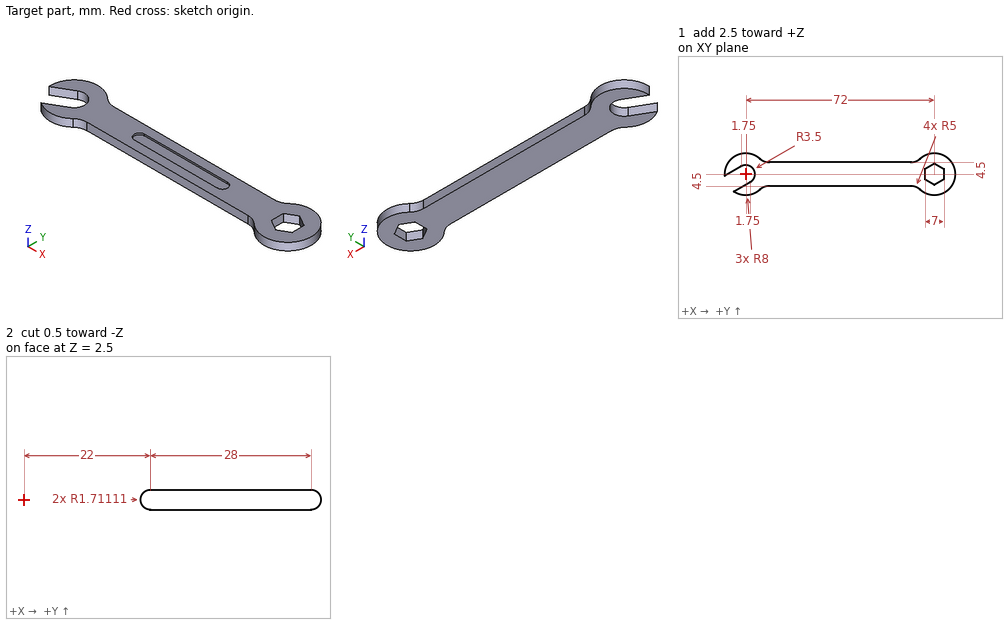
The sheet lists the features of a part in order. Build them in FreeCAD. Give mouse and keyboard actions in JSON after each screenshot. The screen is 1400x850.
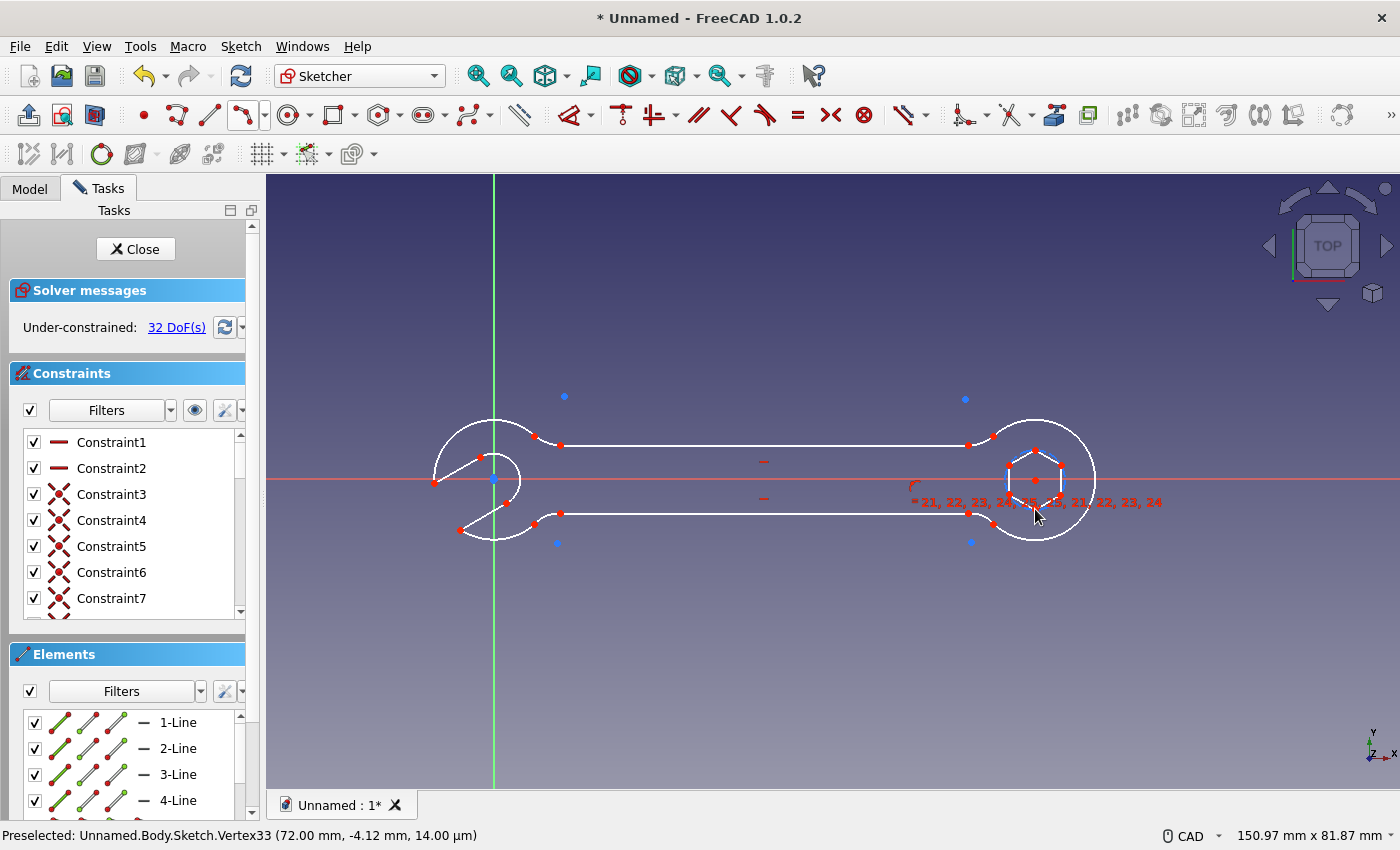
{"action": "left_click", "coordinate": [683, 514]}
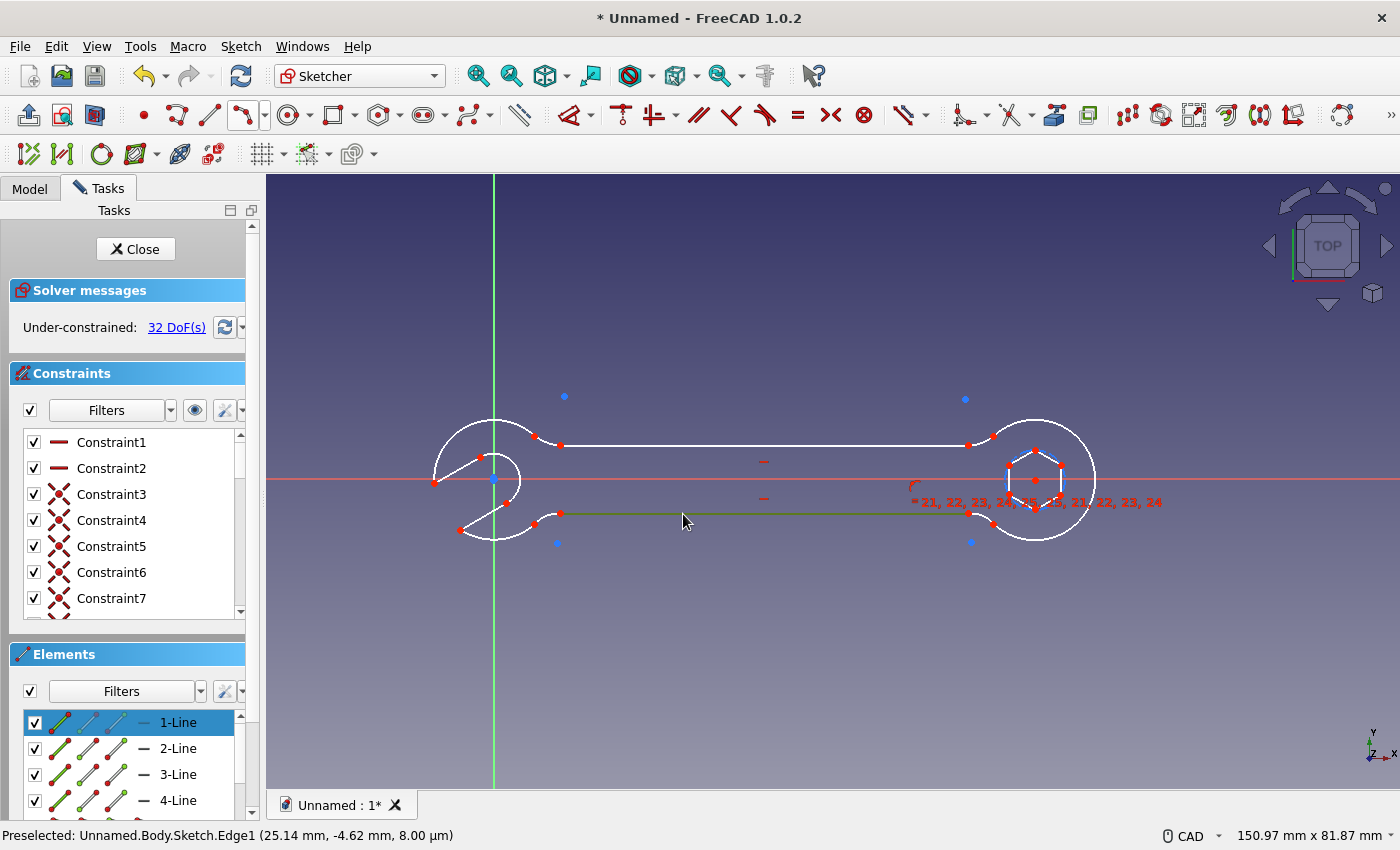
{"action": "left_click", "coordinate": [983, 516]}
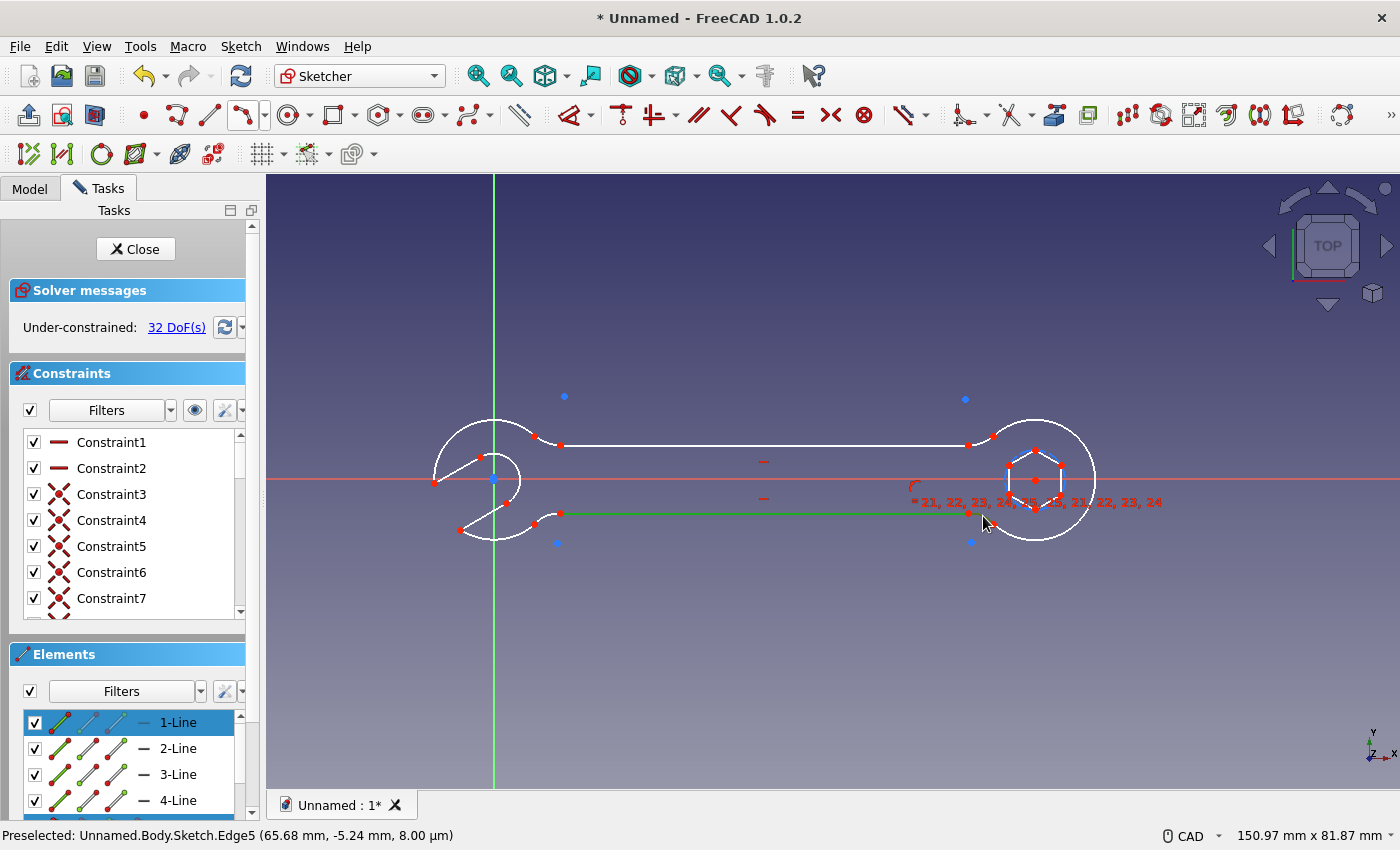
{"action": "key", "text": "t"}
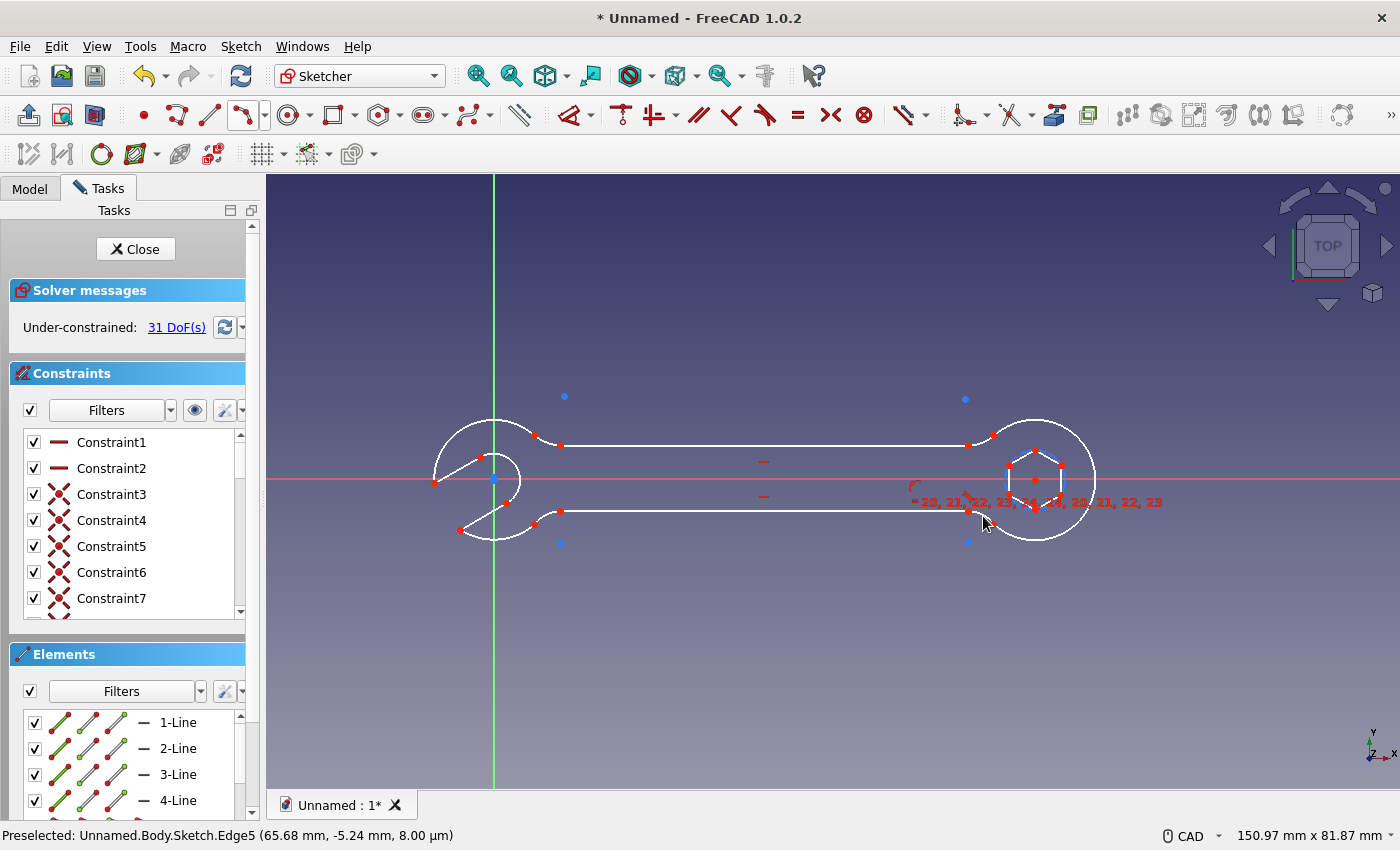
{"action": "left_click", "coordinate": [683, 511]}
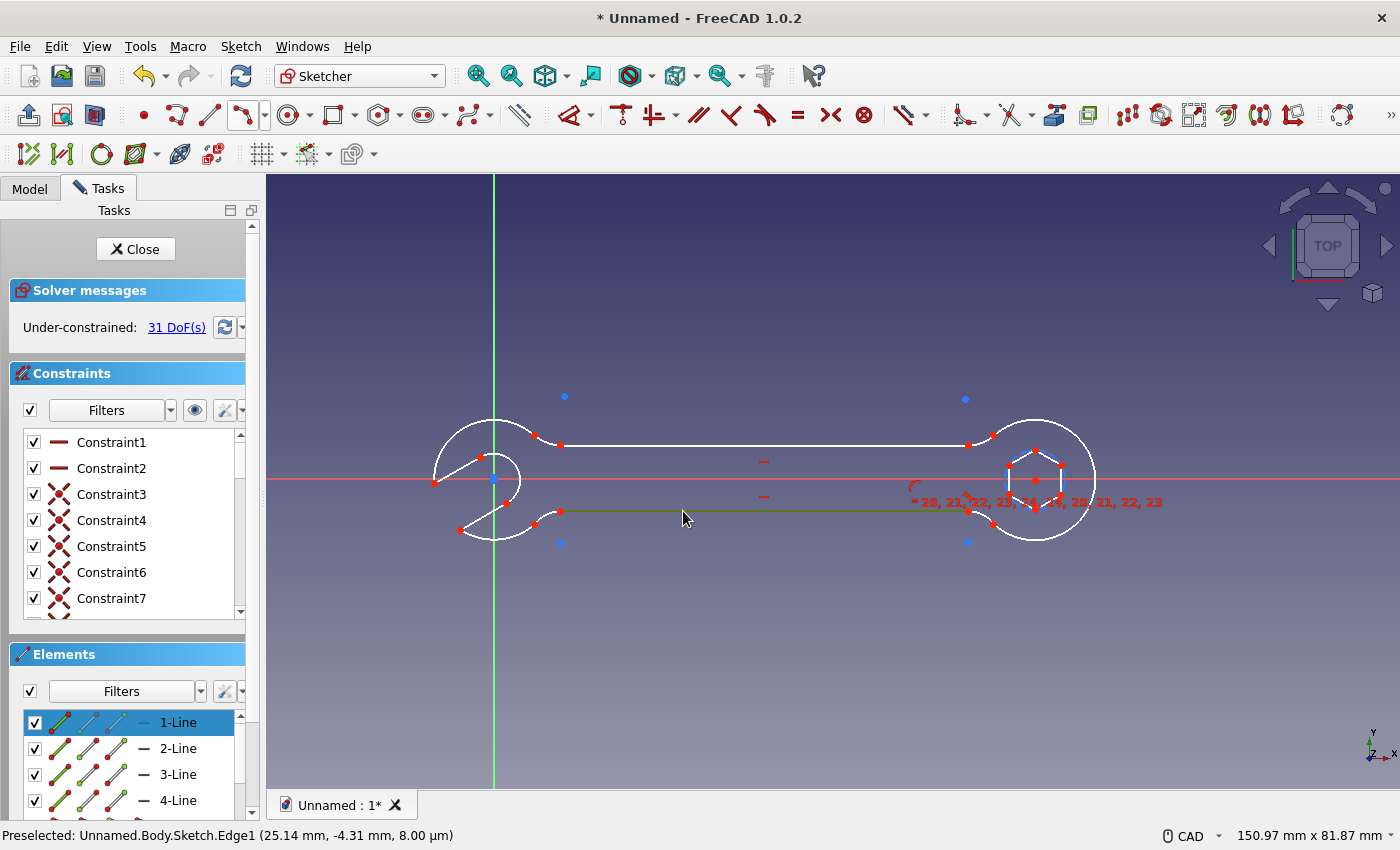
{"action": "left_click", "coordinate": [546, 515]}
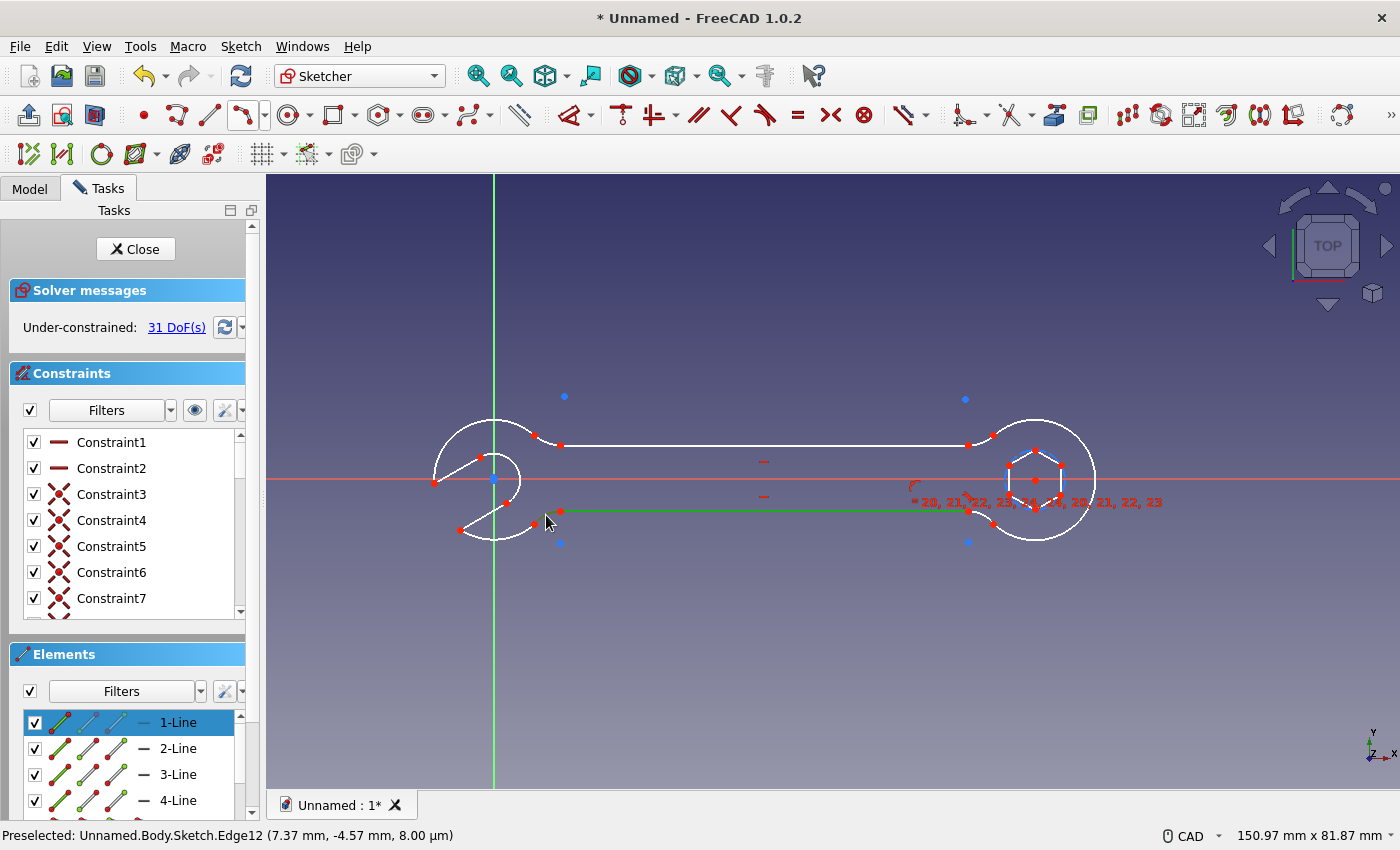
{"action": "left_click", "coordinate": [765, 116]}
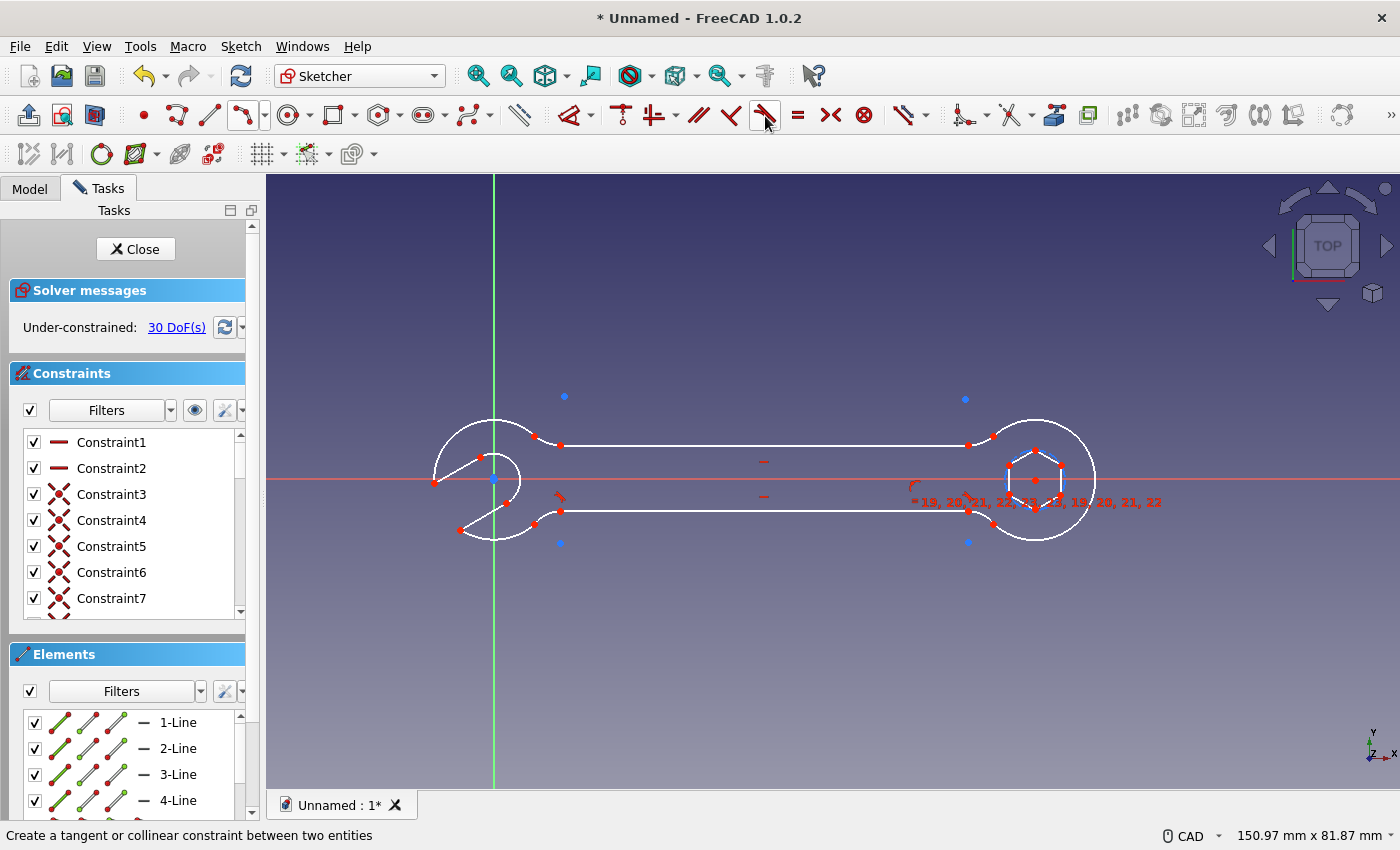
{"action": "left_click", "coordinate": [846, 446]}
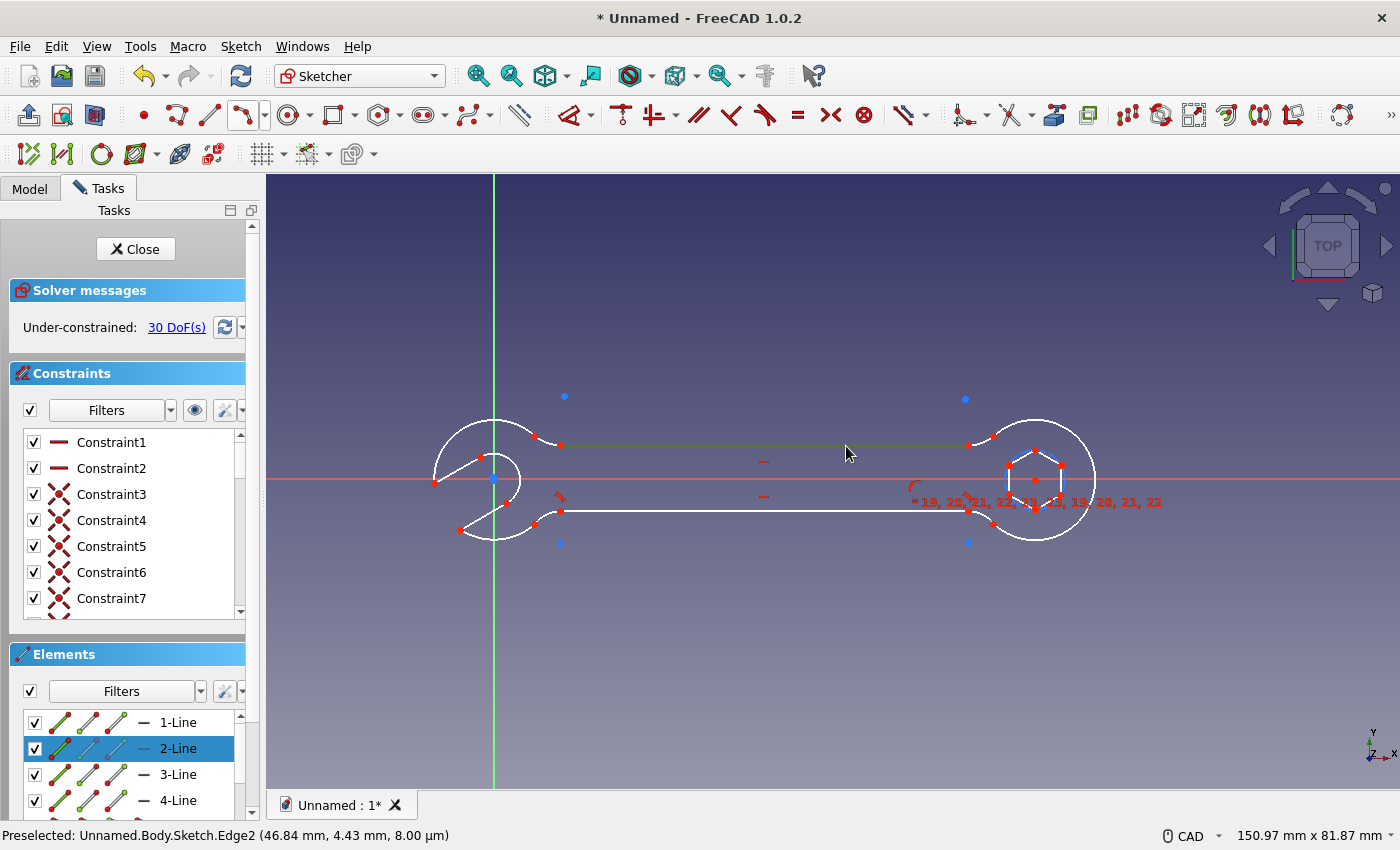
{"action": "left_click", "coordinate": [982, 443]}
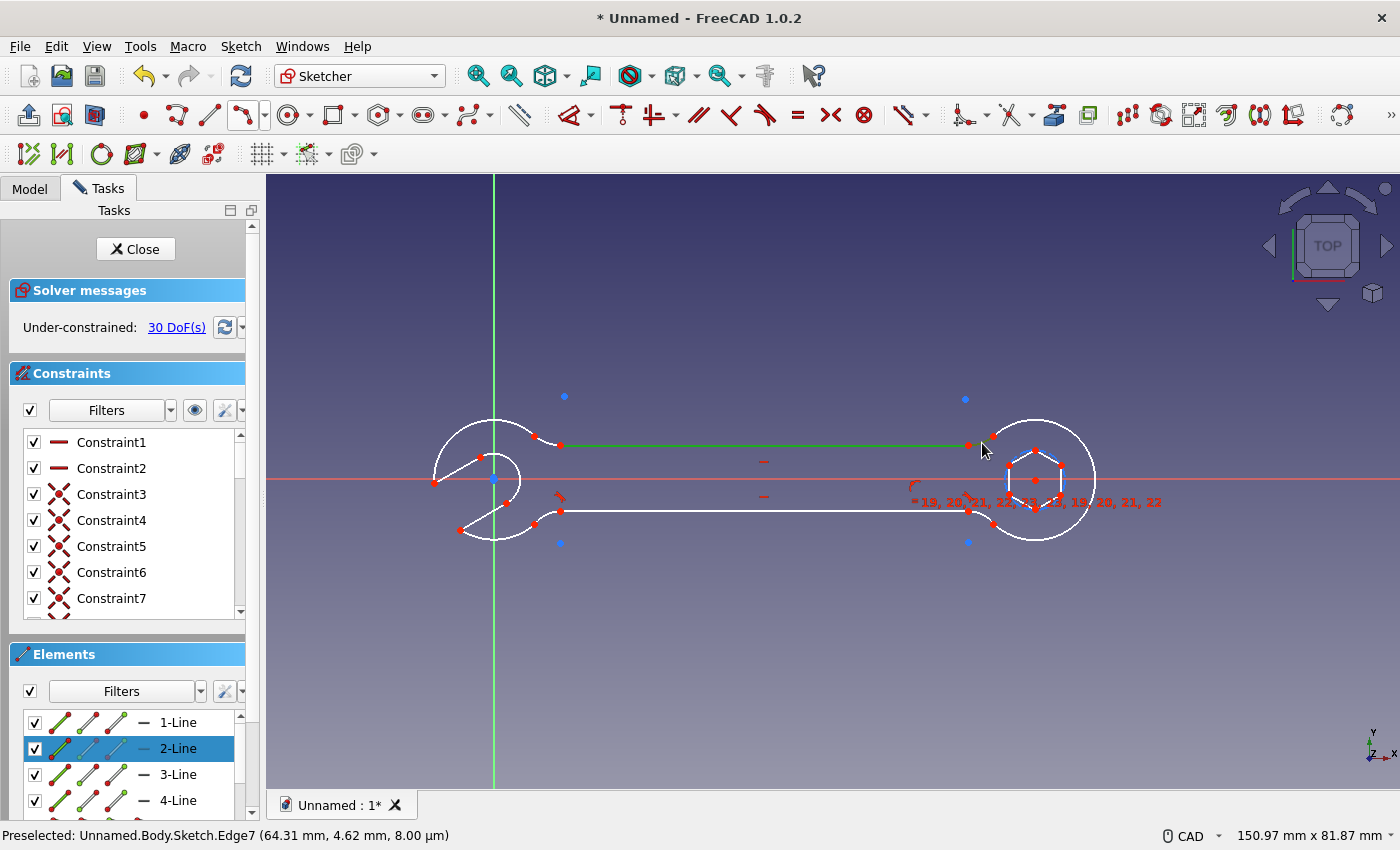
{"action": "left_click", "coordinate": [765, 116]}